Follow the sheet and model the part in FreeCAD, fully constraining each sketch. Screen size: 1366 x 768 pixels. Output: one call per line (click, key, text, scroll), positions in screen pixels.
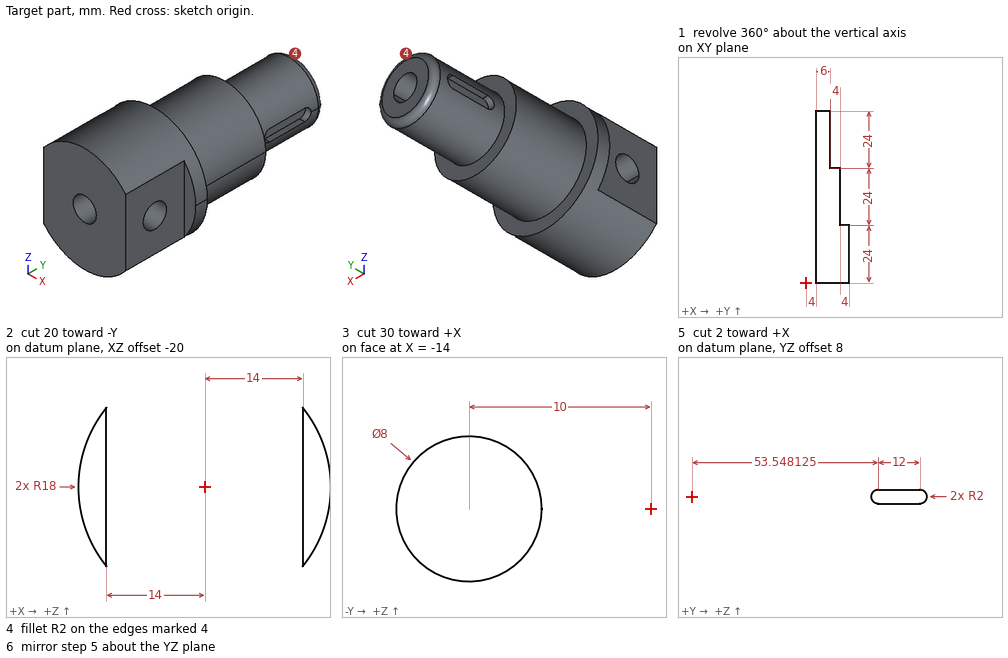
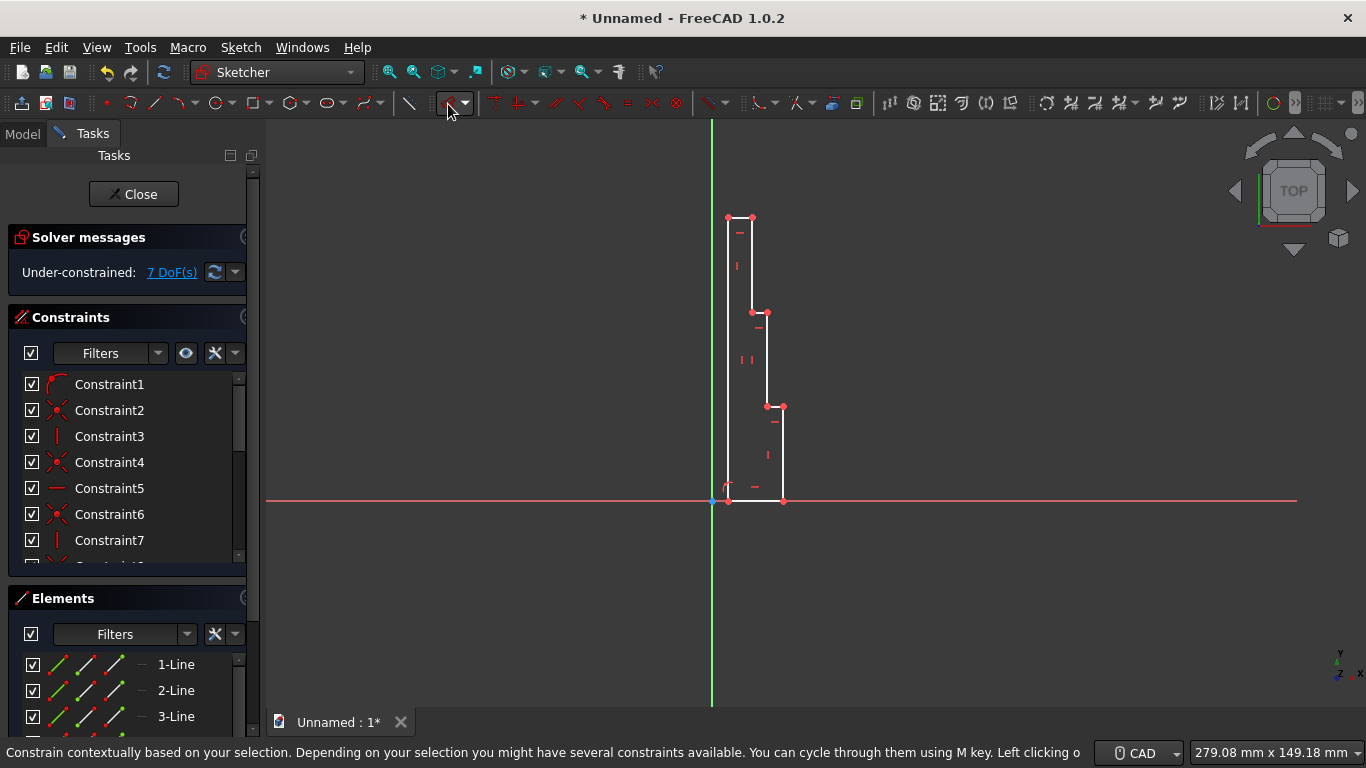
scroll(775, 407, up, 5)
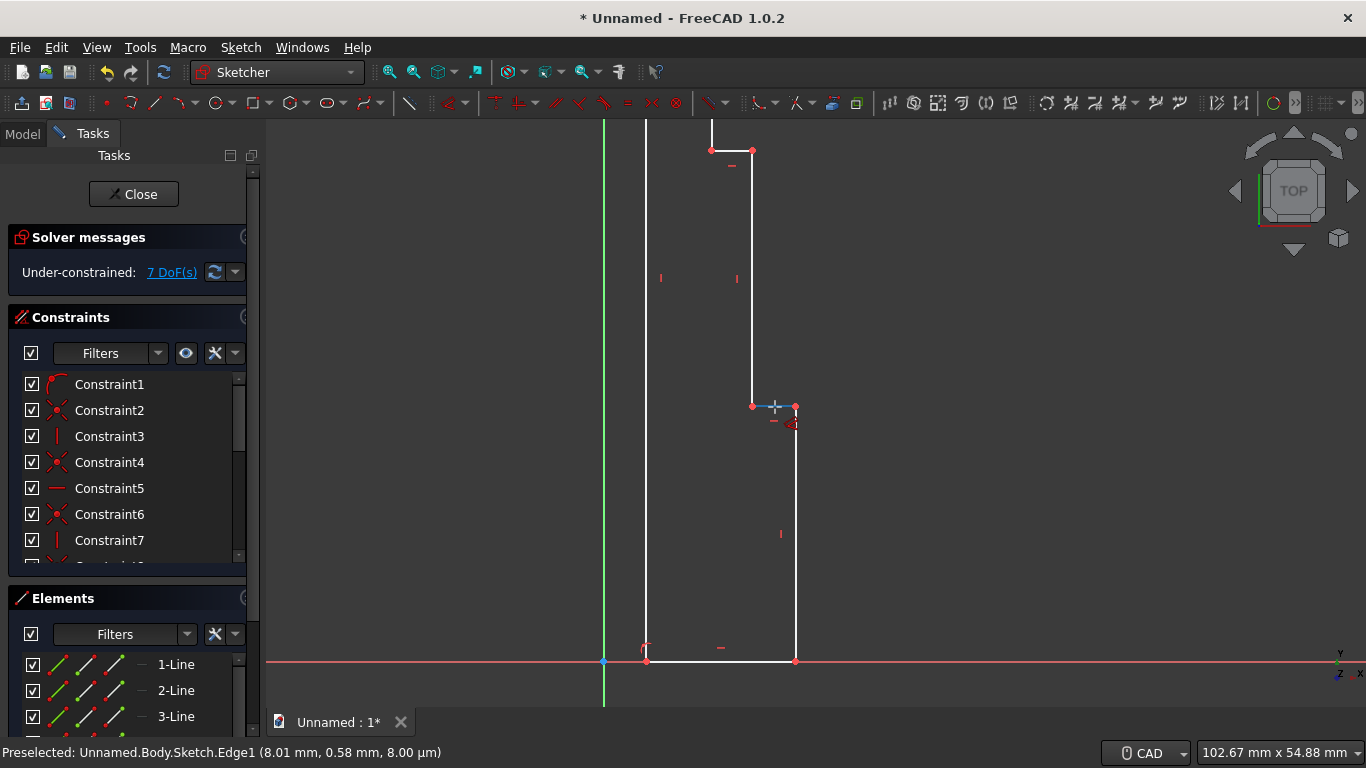
click(774, 406)
click(774, 440)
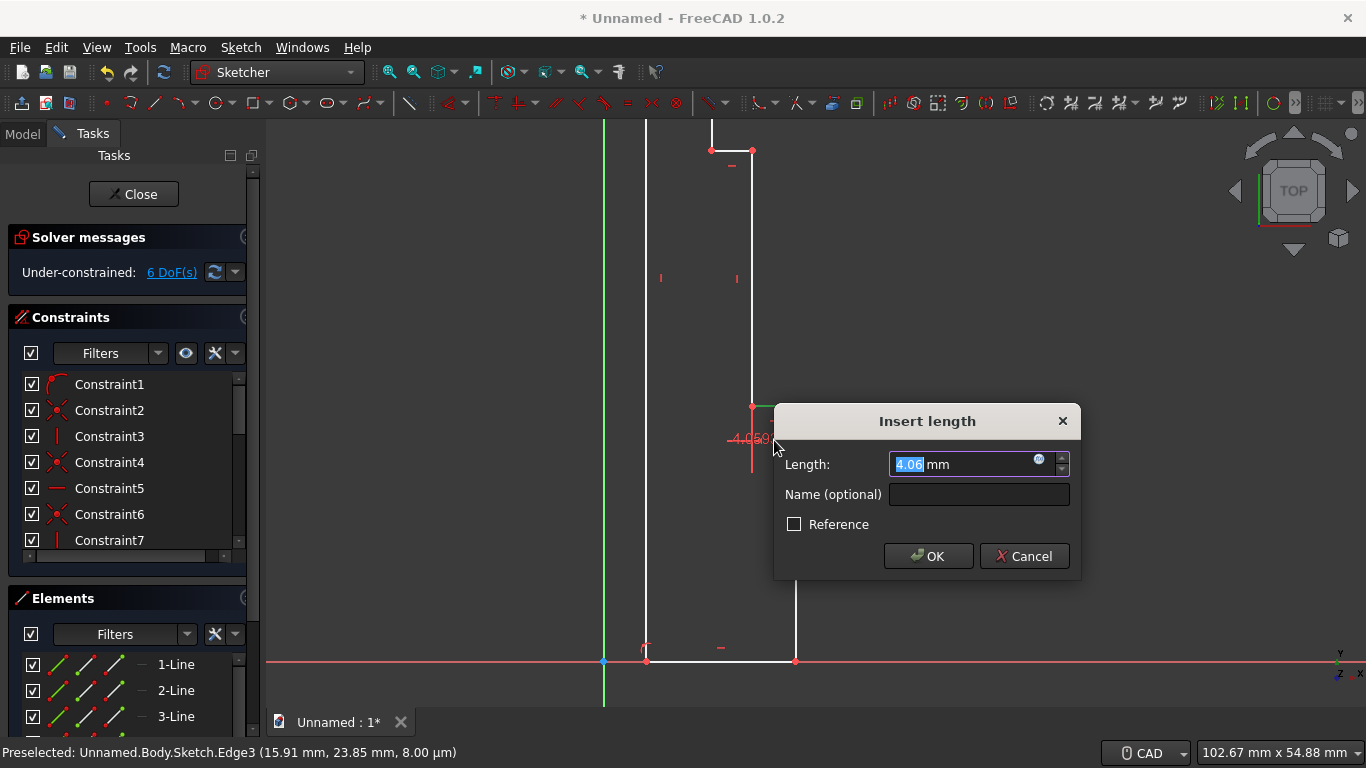
text(4)
key(Return)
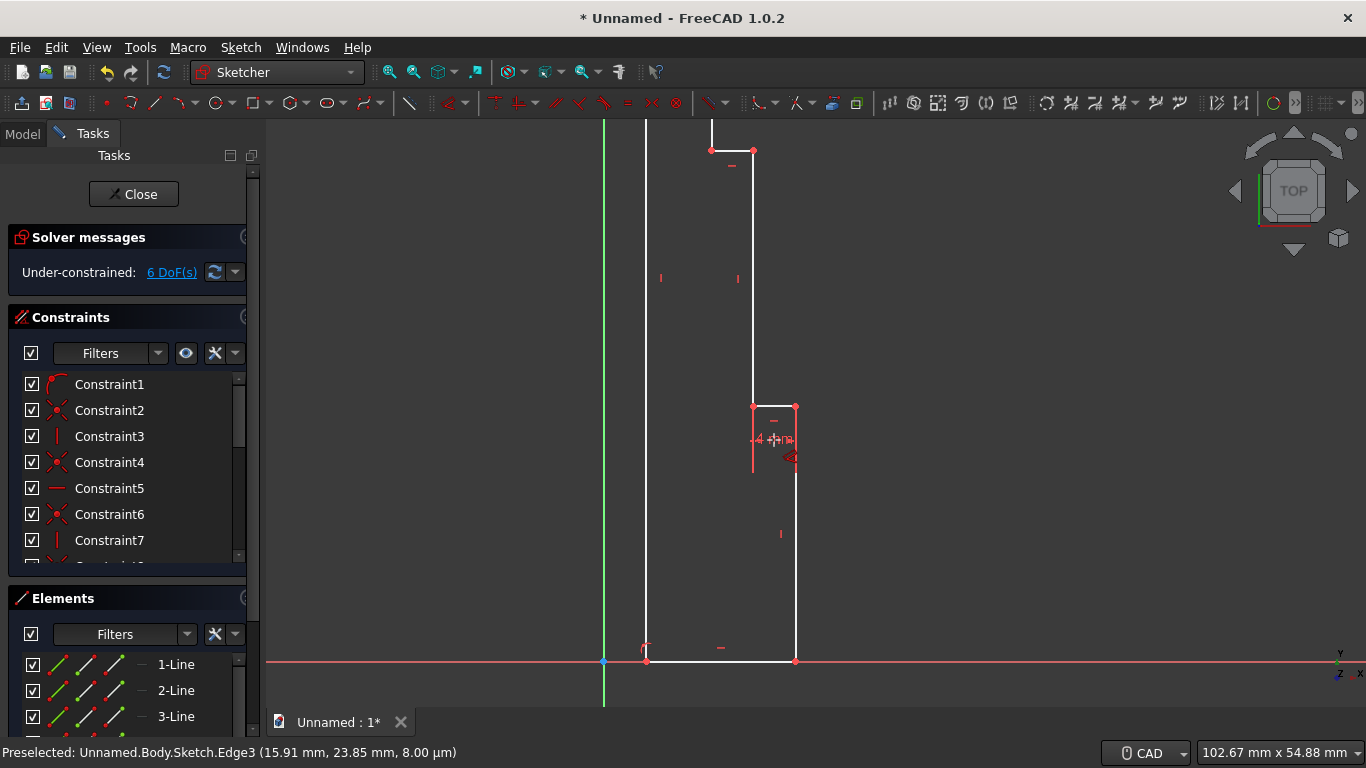
click(741, 151)
click(732, 185)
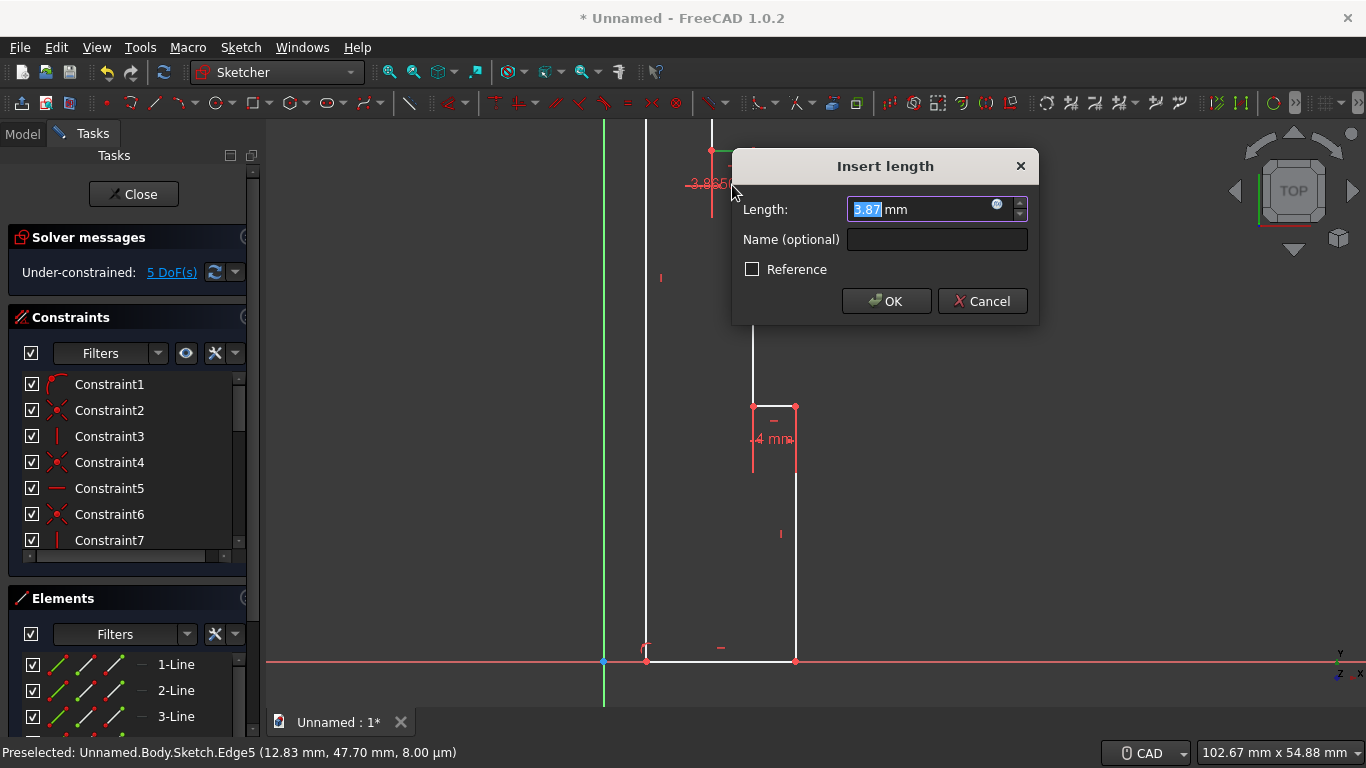
text(4)
key(Return)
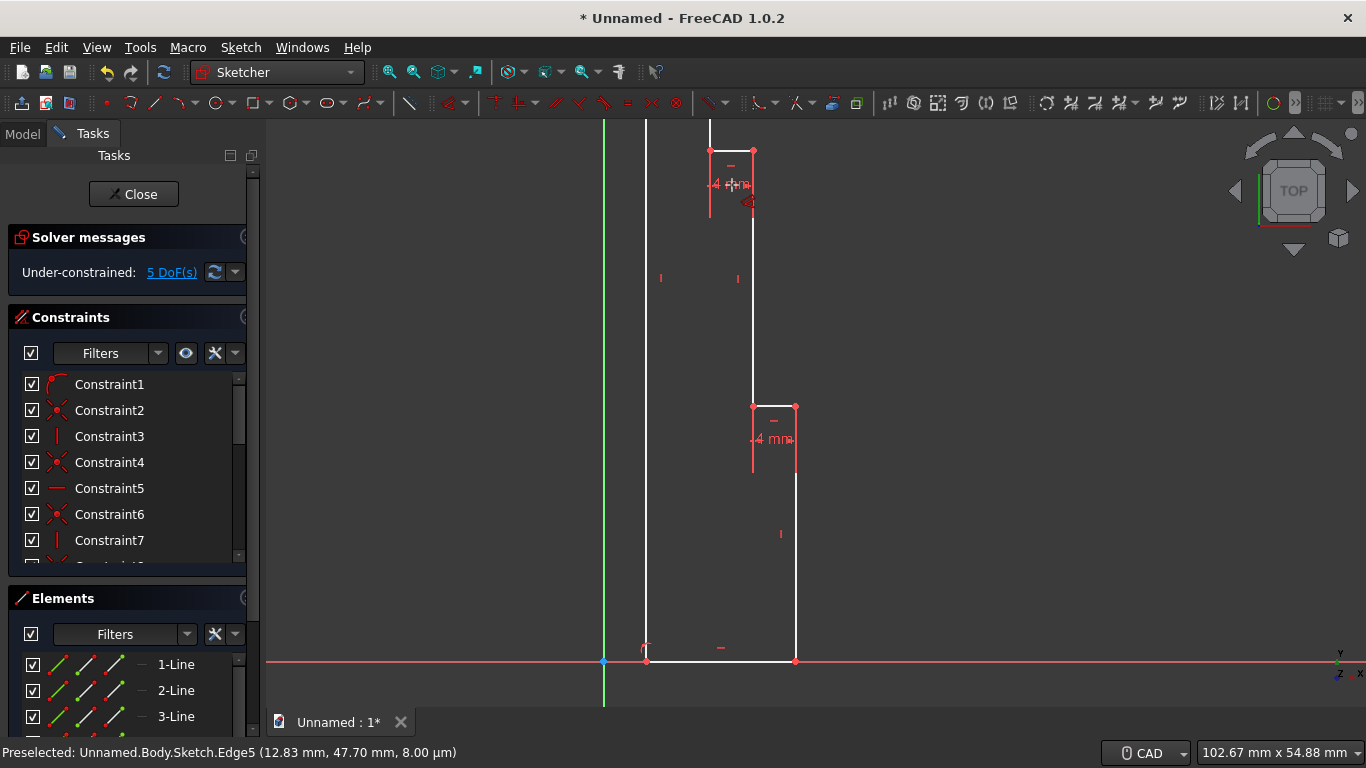
scroll(786, 525, down, 4)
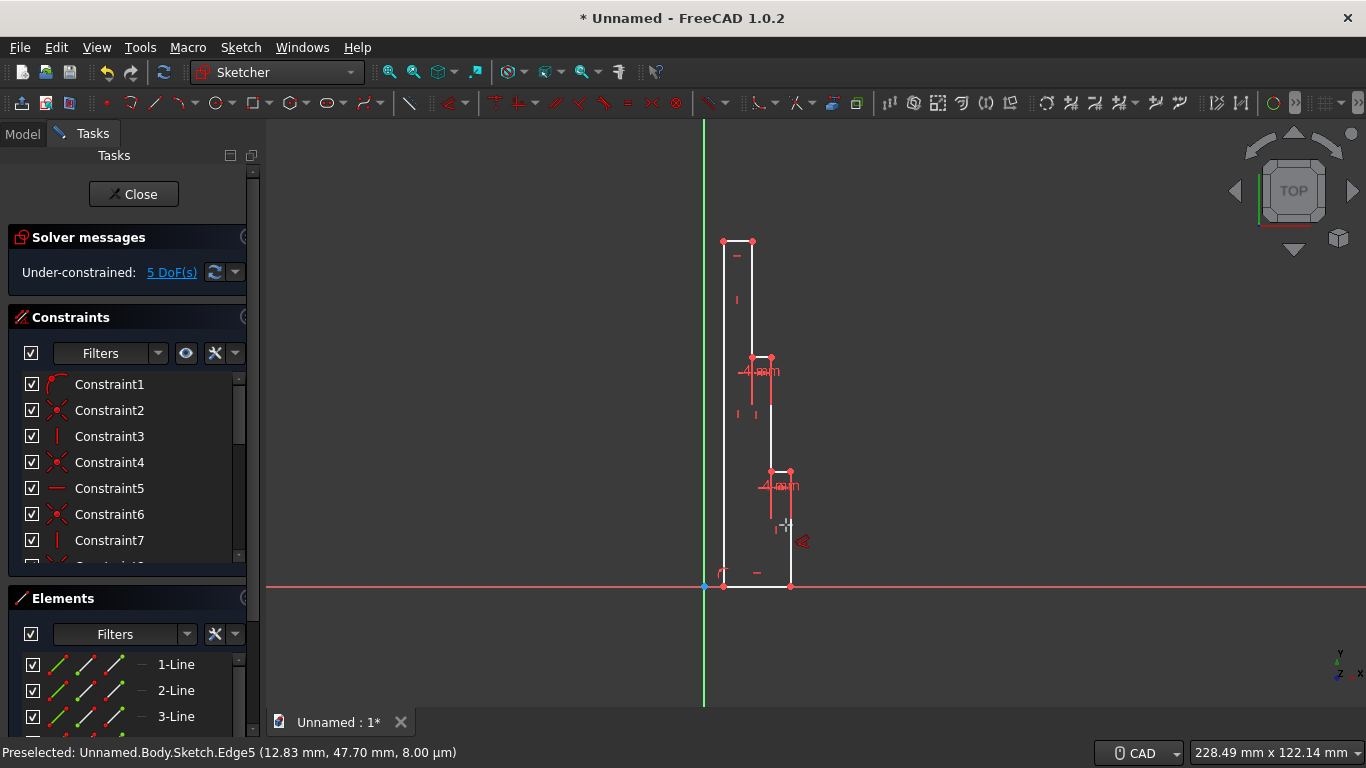
scroll(744, 241, up, 3)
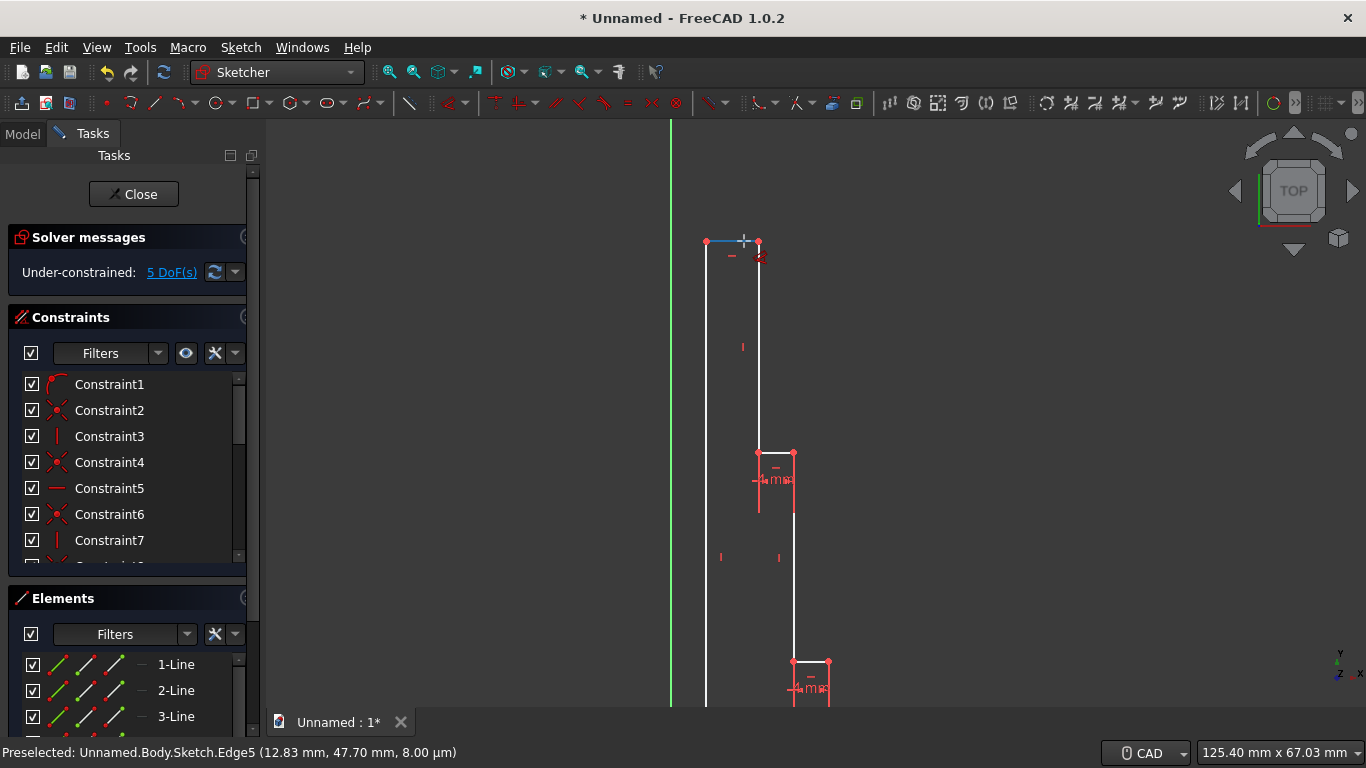
click(743, 241)
click(733, 207)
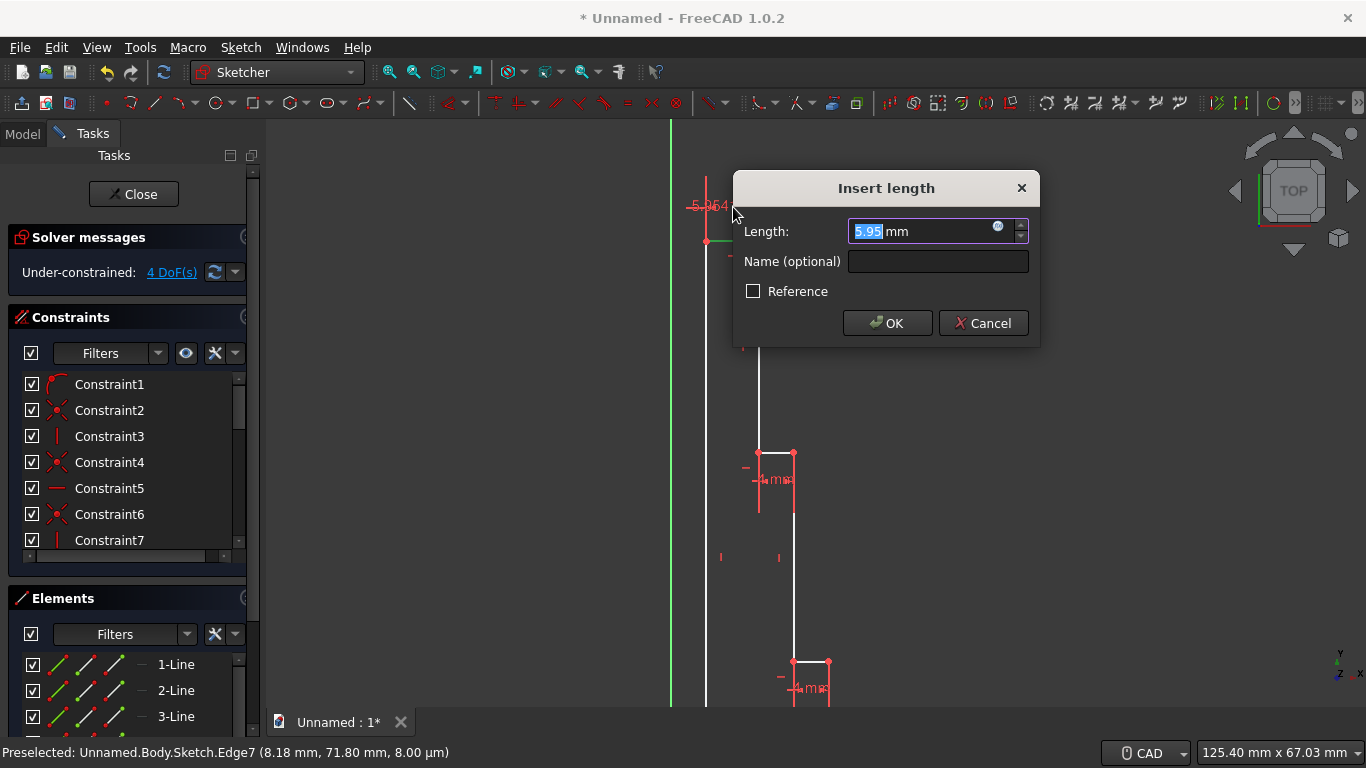
text(6)
key(Return)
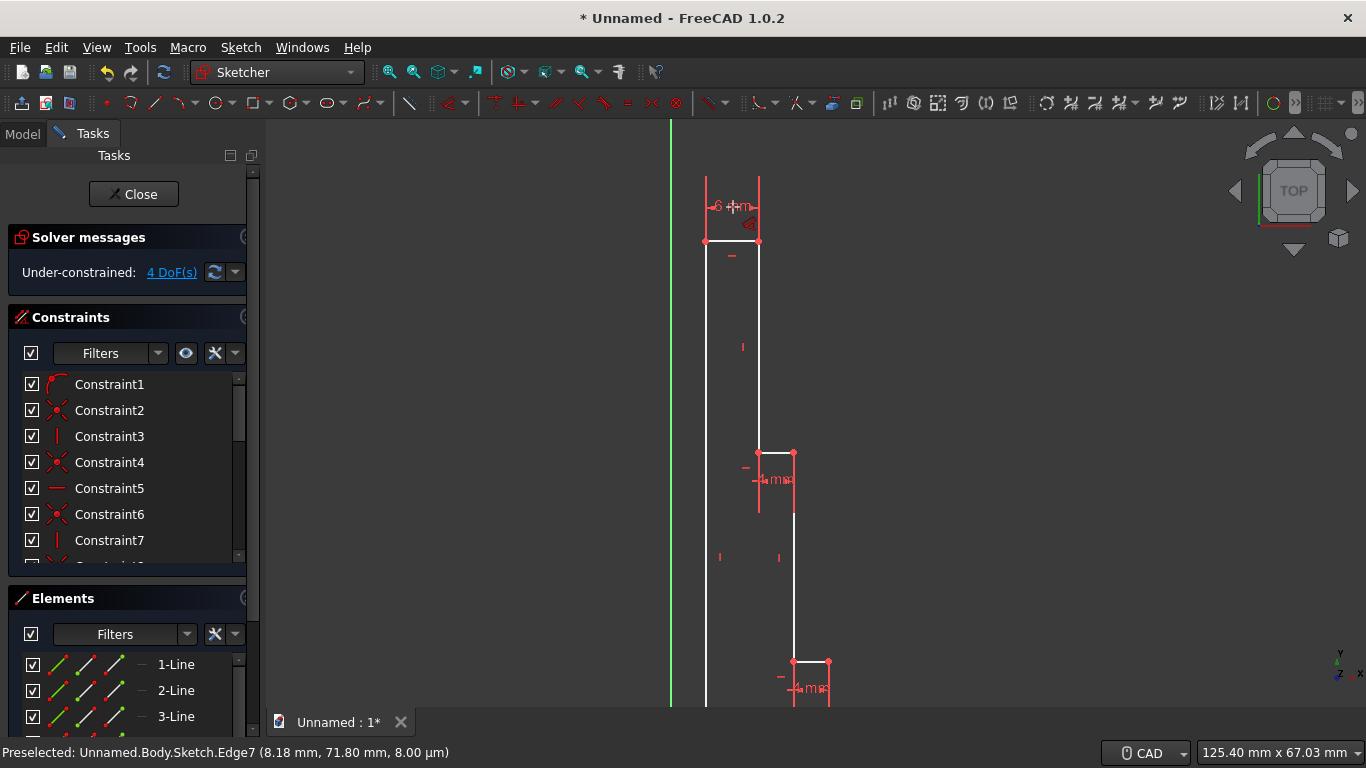
scroll(744, 240, down, 3)